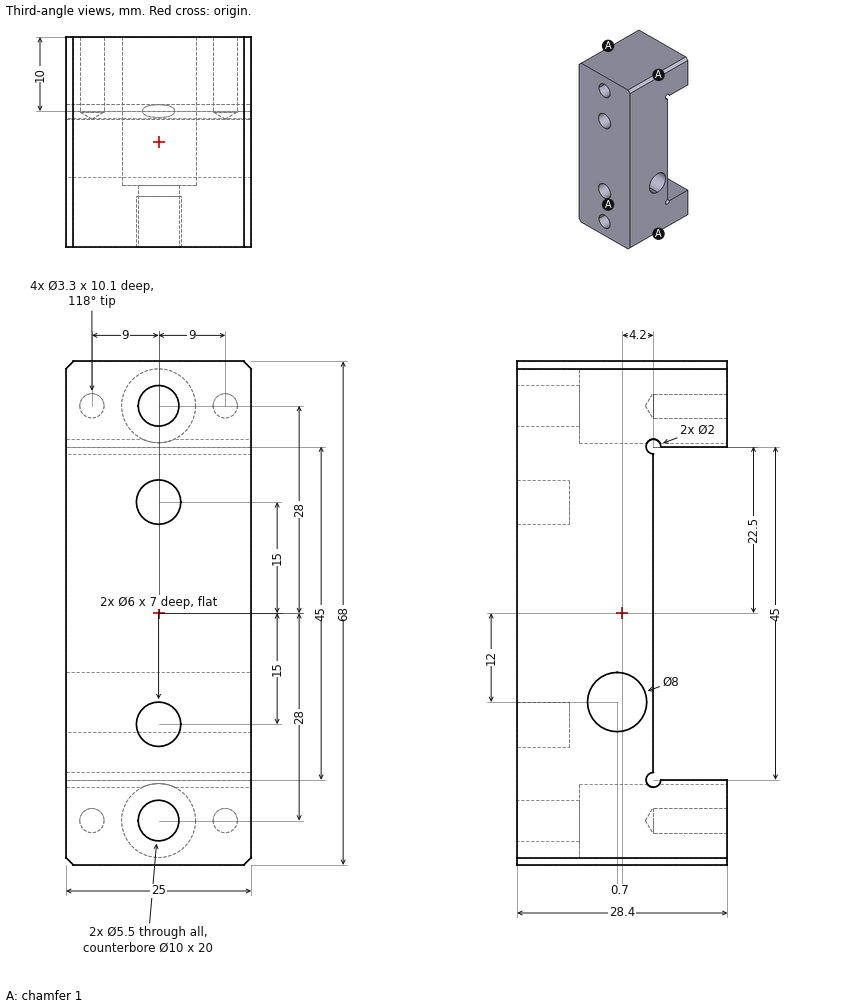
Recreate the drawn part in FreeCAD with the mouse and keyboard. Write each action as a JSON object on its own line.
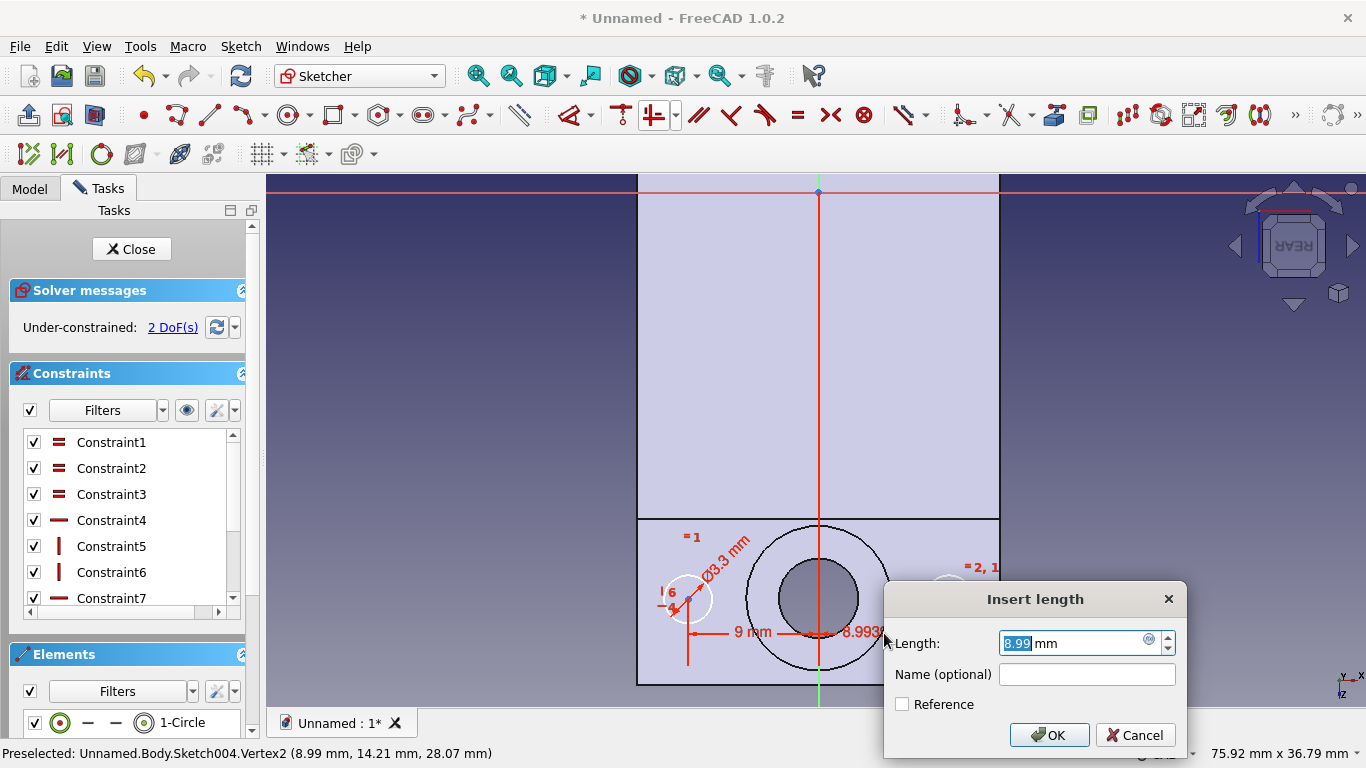
{"action": "type", "text": "9"}
{"action": "key", "text": "Return"}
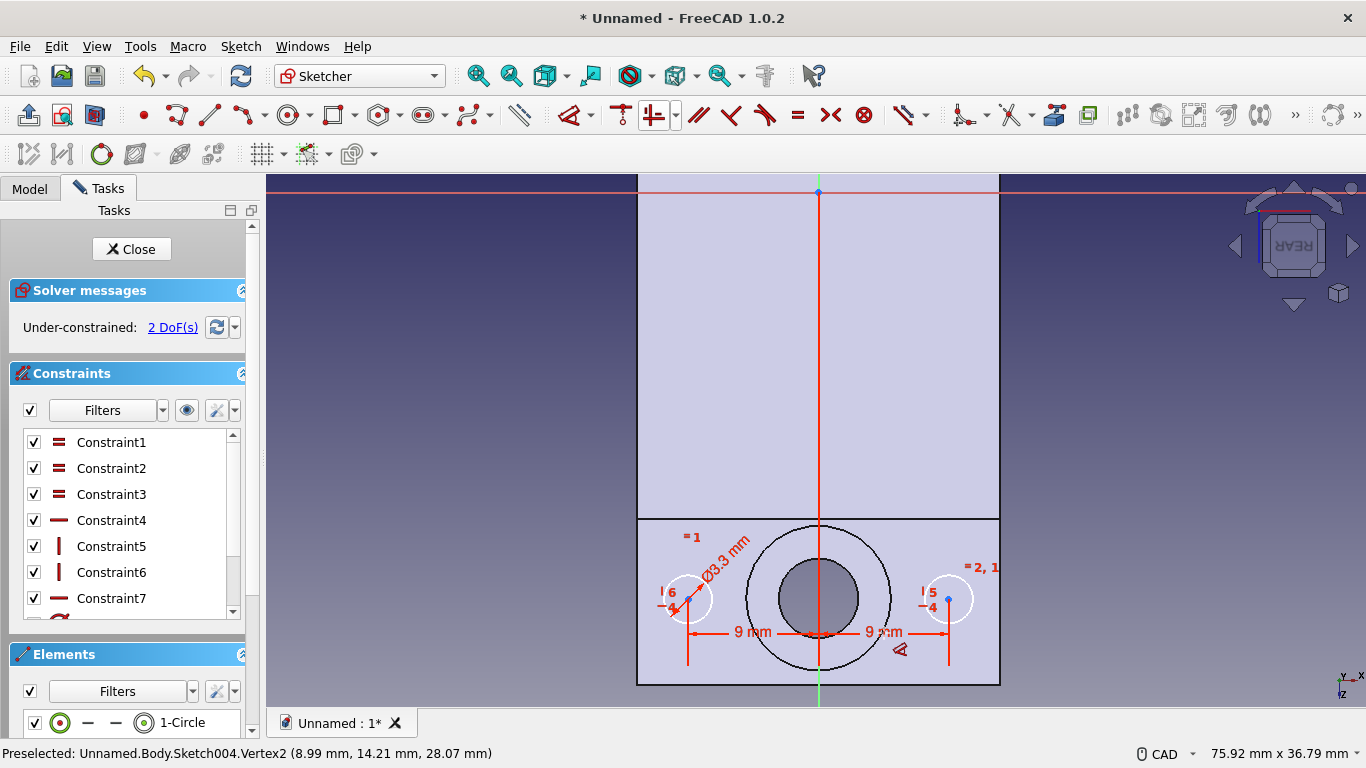
{"action": "left_click", "coordinate": [688, 599]}
{"action": "left_click", "coordinate": [654, 401]}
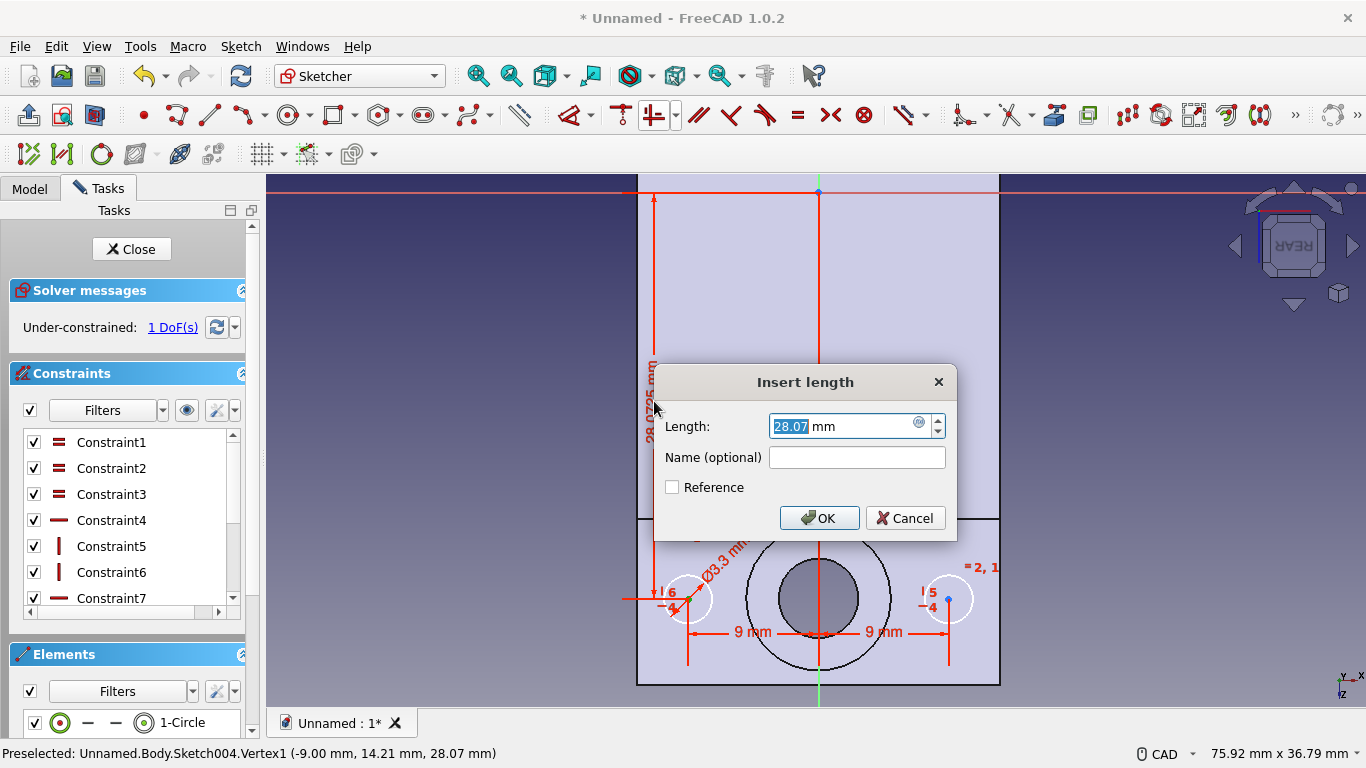
{"action": "type", "text": "28"}
{"action": "key", "text": "Return"}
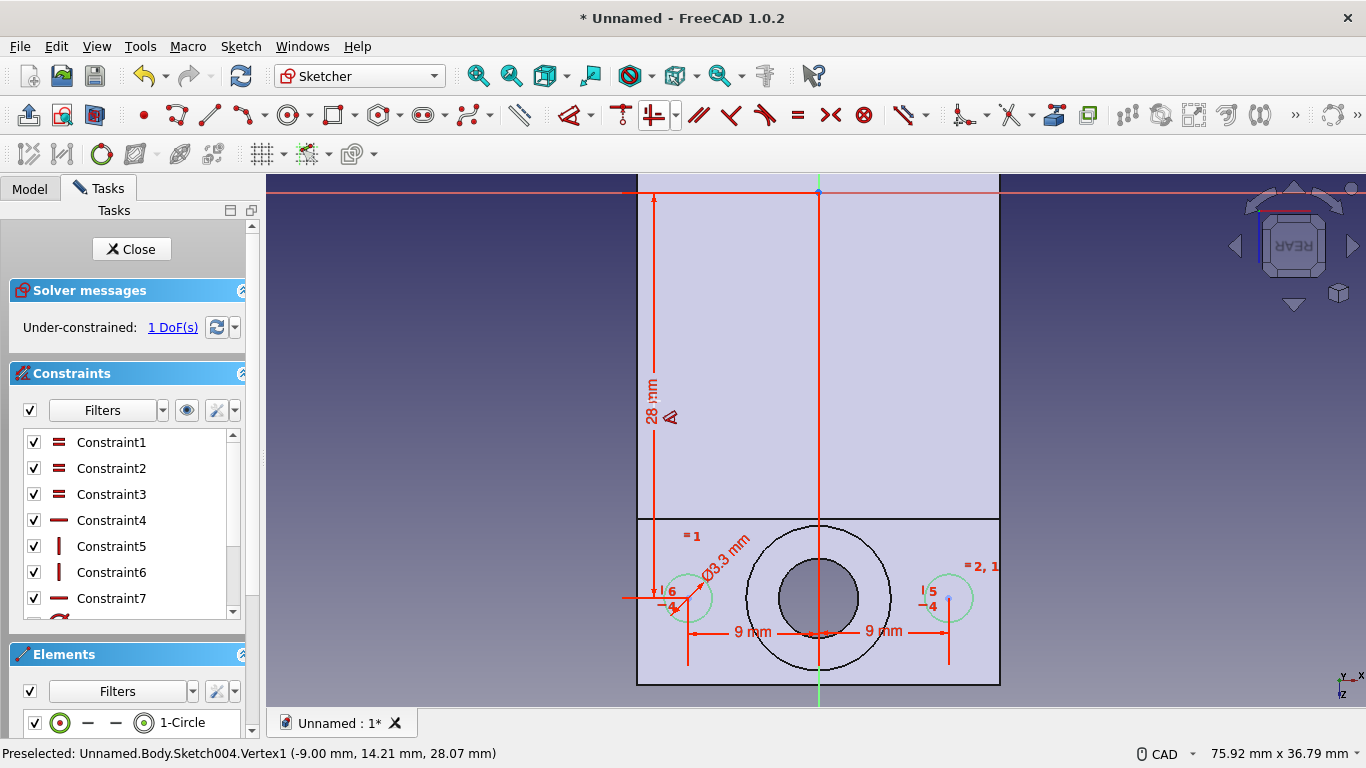
{"action": "scroll", "coordinate": [706, 585], "scroll_direction": "down", "scroll_amount": 5}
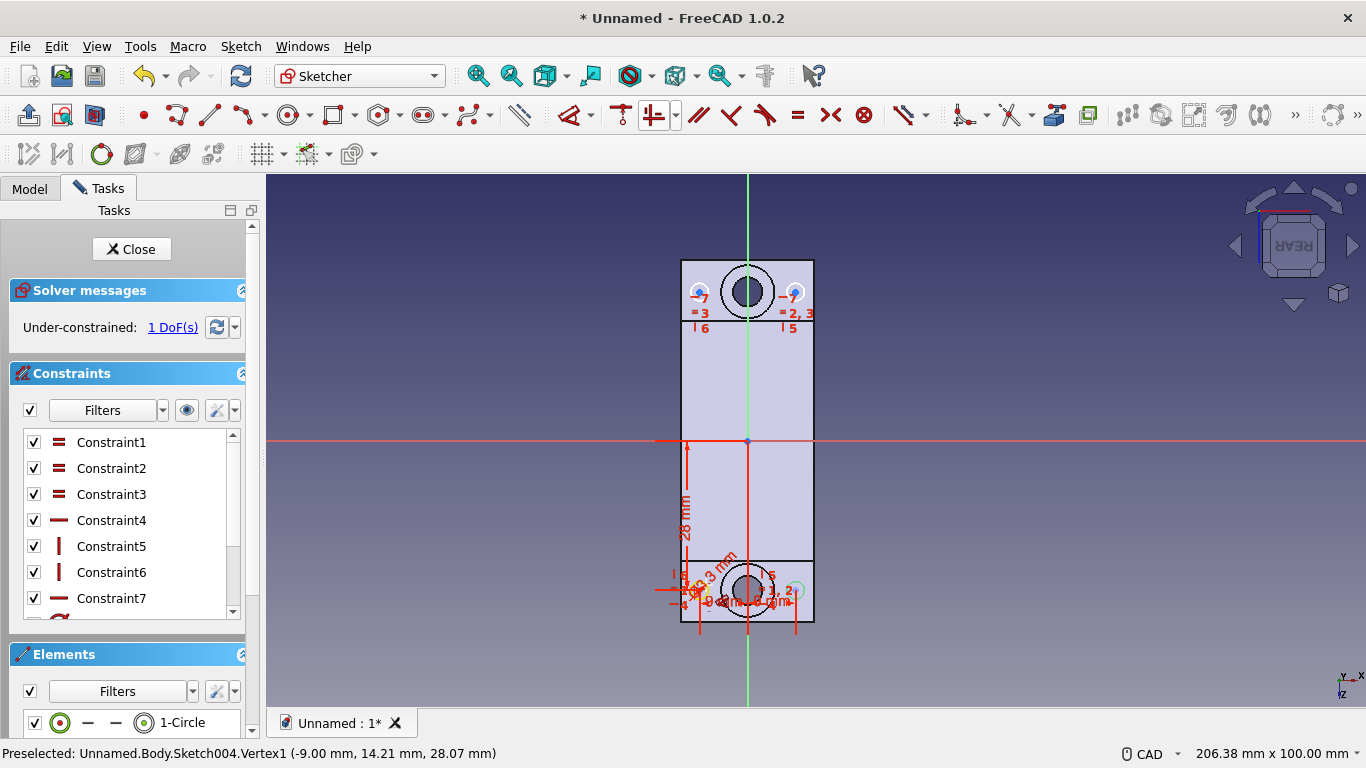
{"action": "left_click", "coordinate": [796, 292]}
{"action": "left_click", "coordinate": [830, 367]}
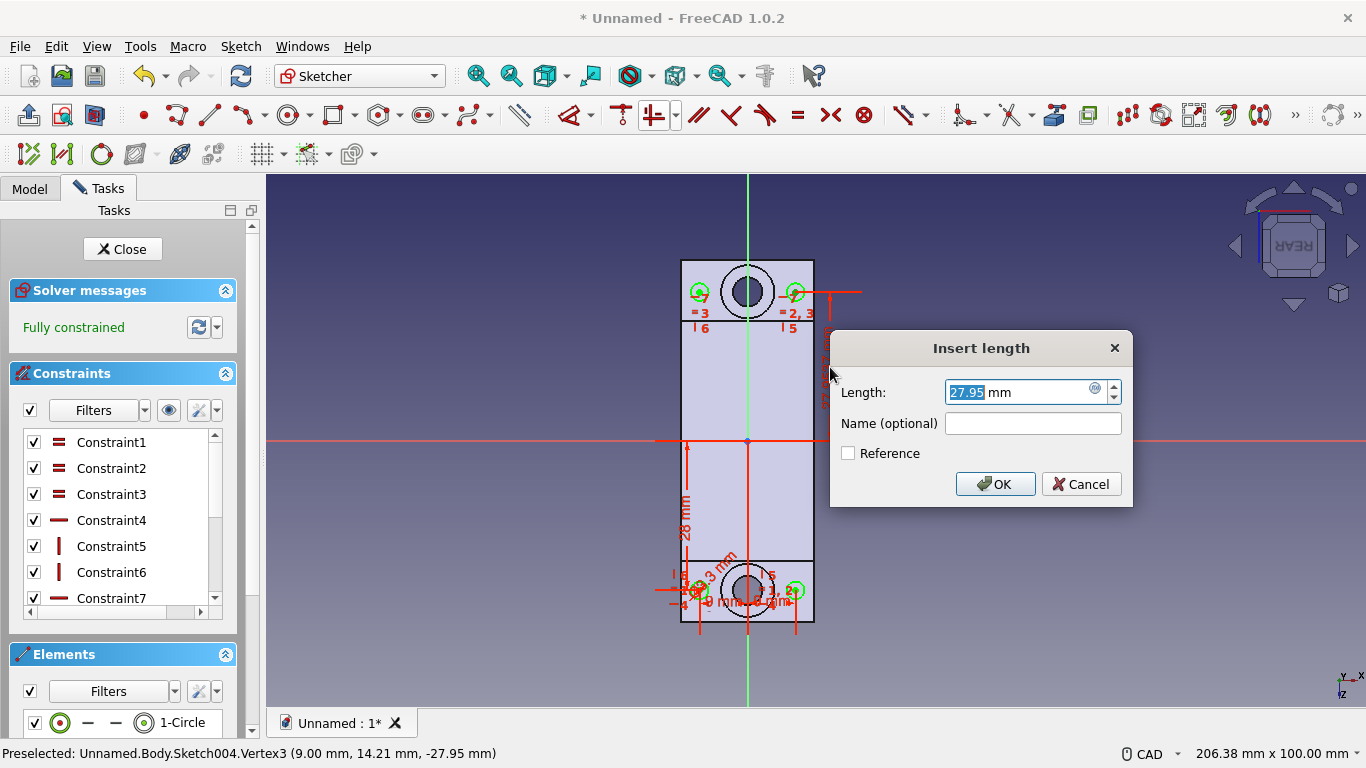
{"action": "type", "text": "28"}
{"action": "key", "text": "Return"}
{"action": "key", "text": "Escape"}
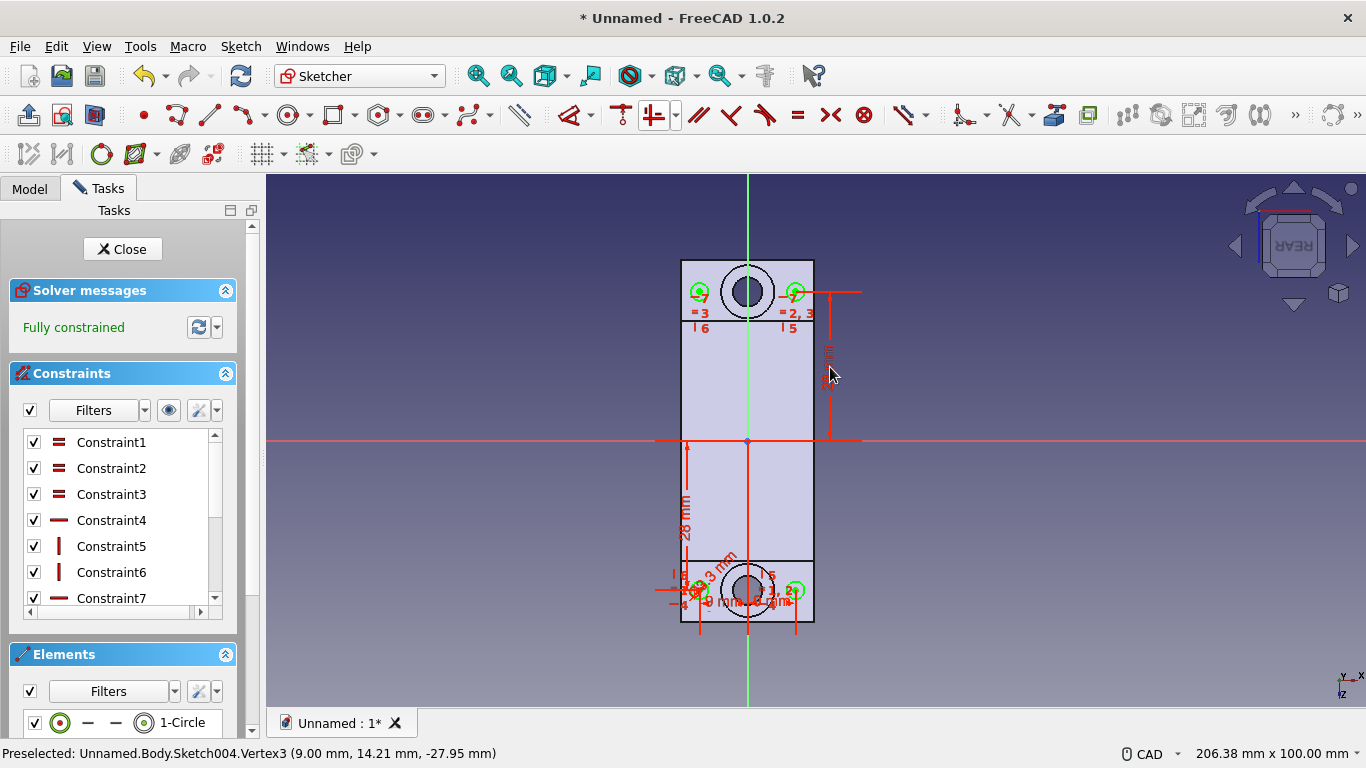
{"action": "left_click", "coordinate": [123, 249]}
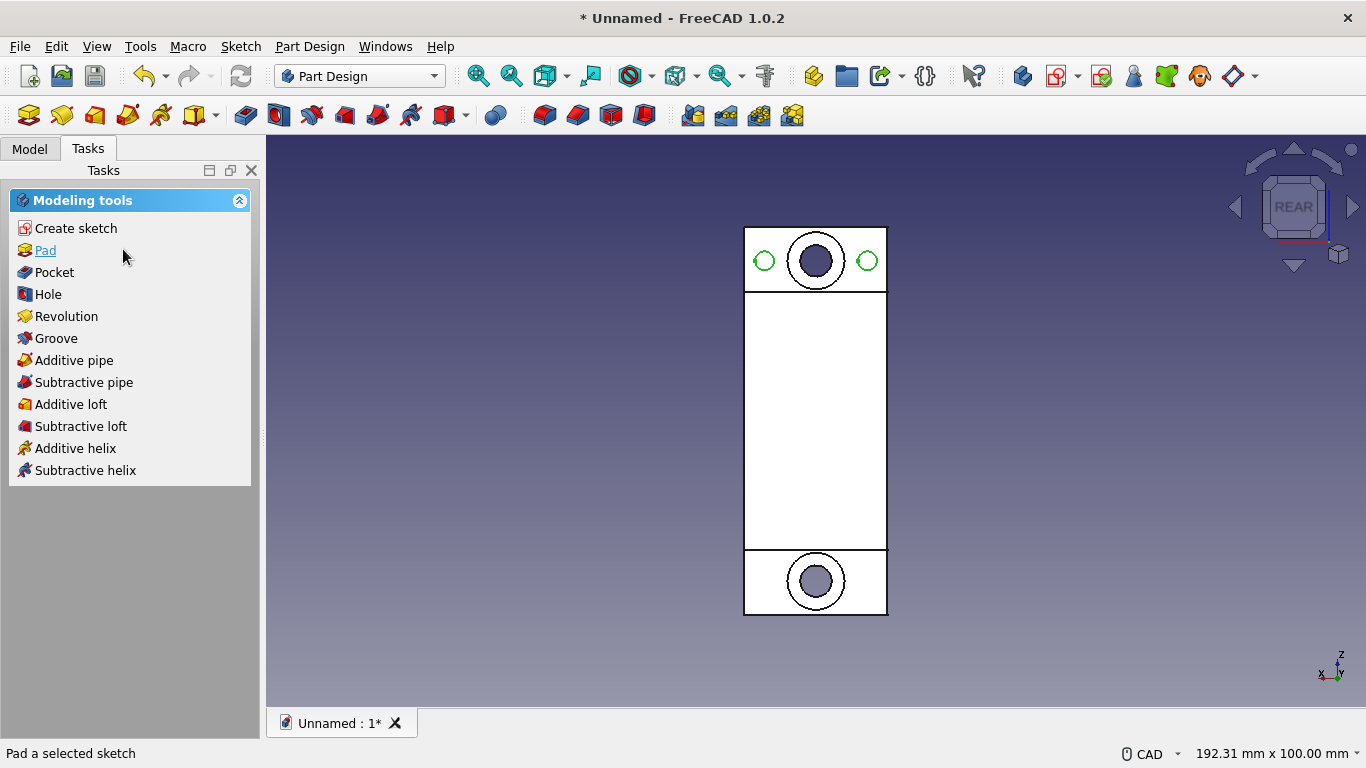
{"action": "left_click", "coordinate": [279, 116]}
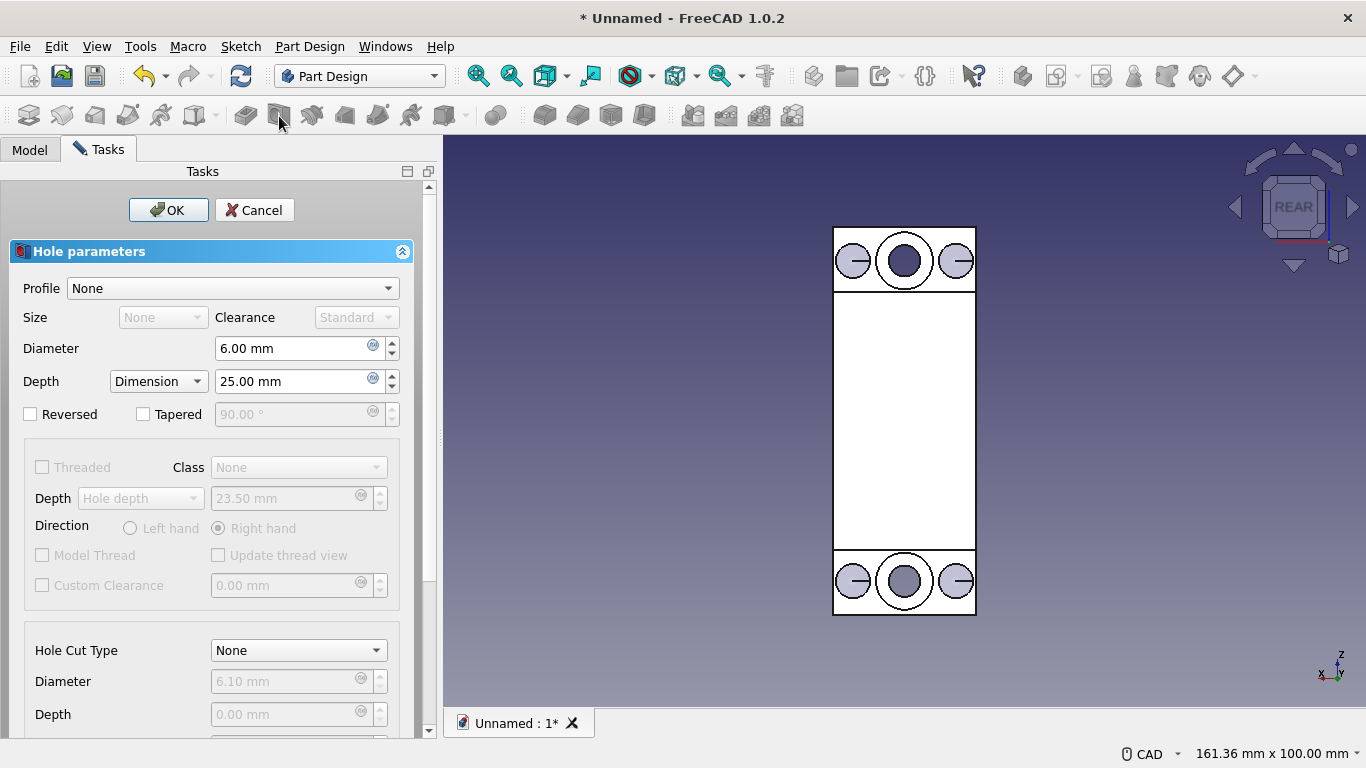
{"action": "triple_click", "coordinate": [300, 348]}